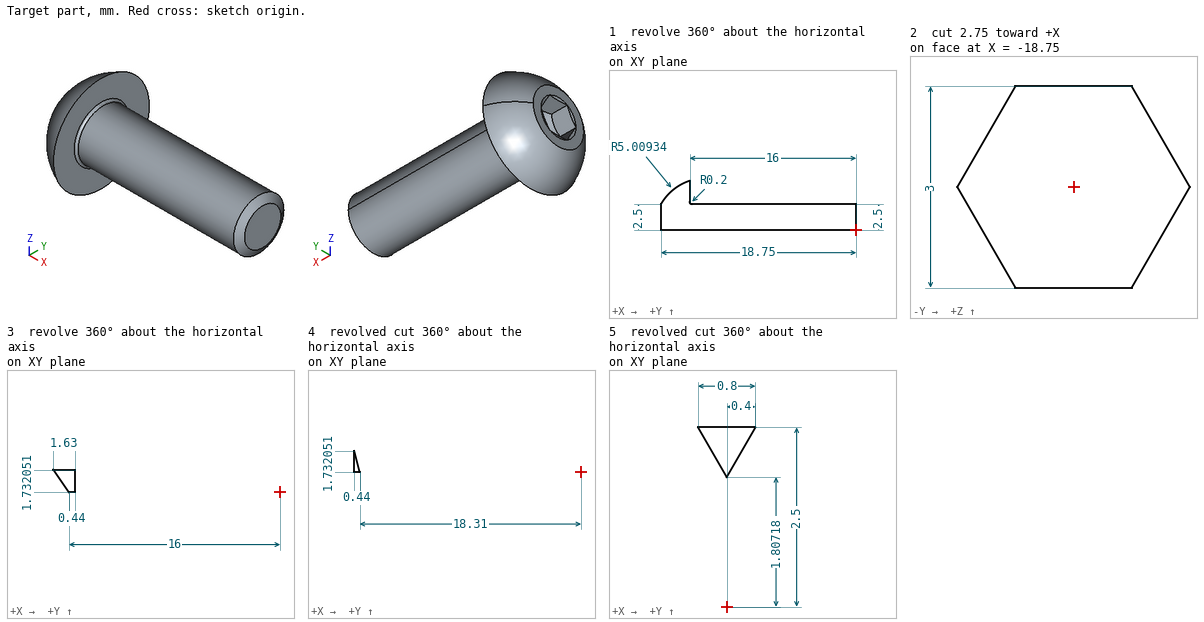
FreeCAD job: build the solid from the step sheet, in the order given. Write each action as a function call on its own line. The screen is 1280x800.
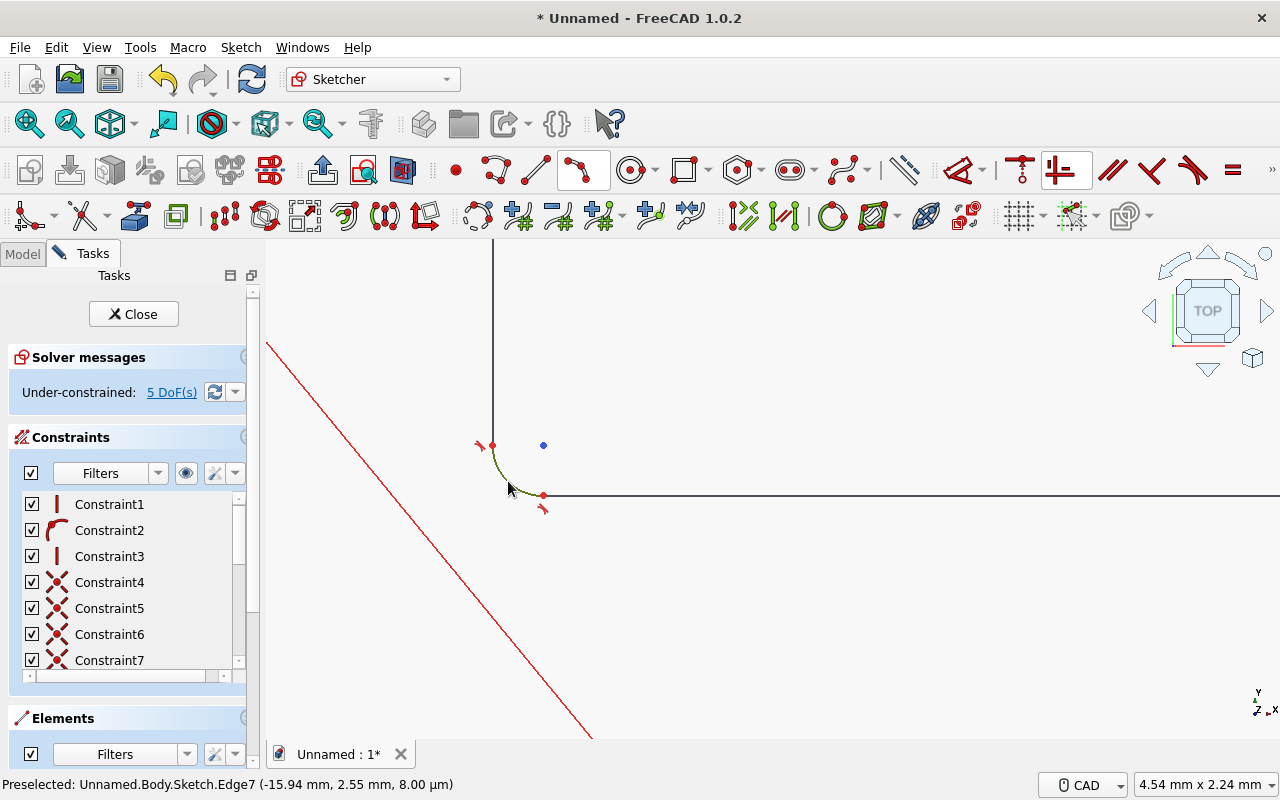
key(k)
key(r)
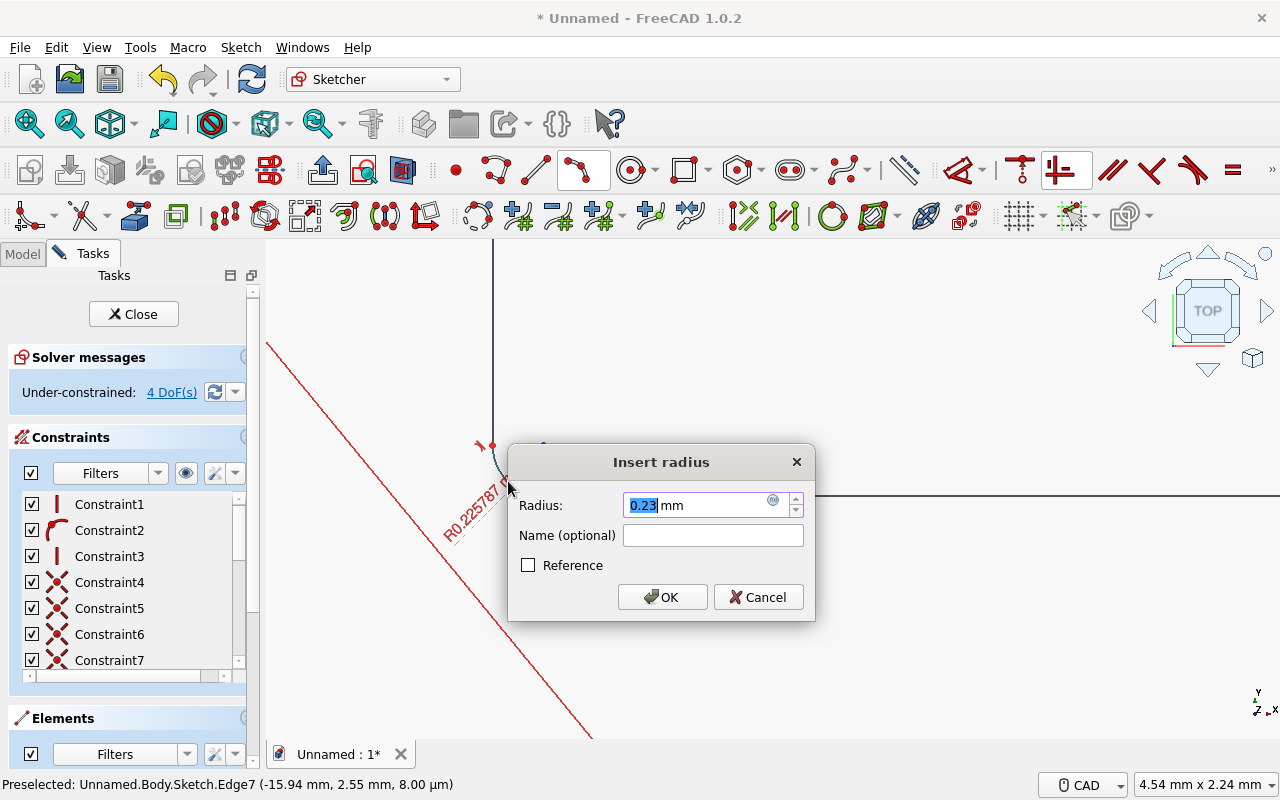
text(0.2)
key(Return)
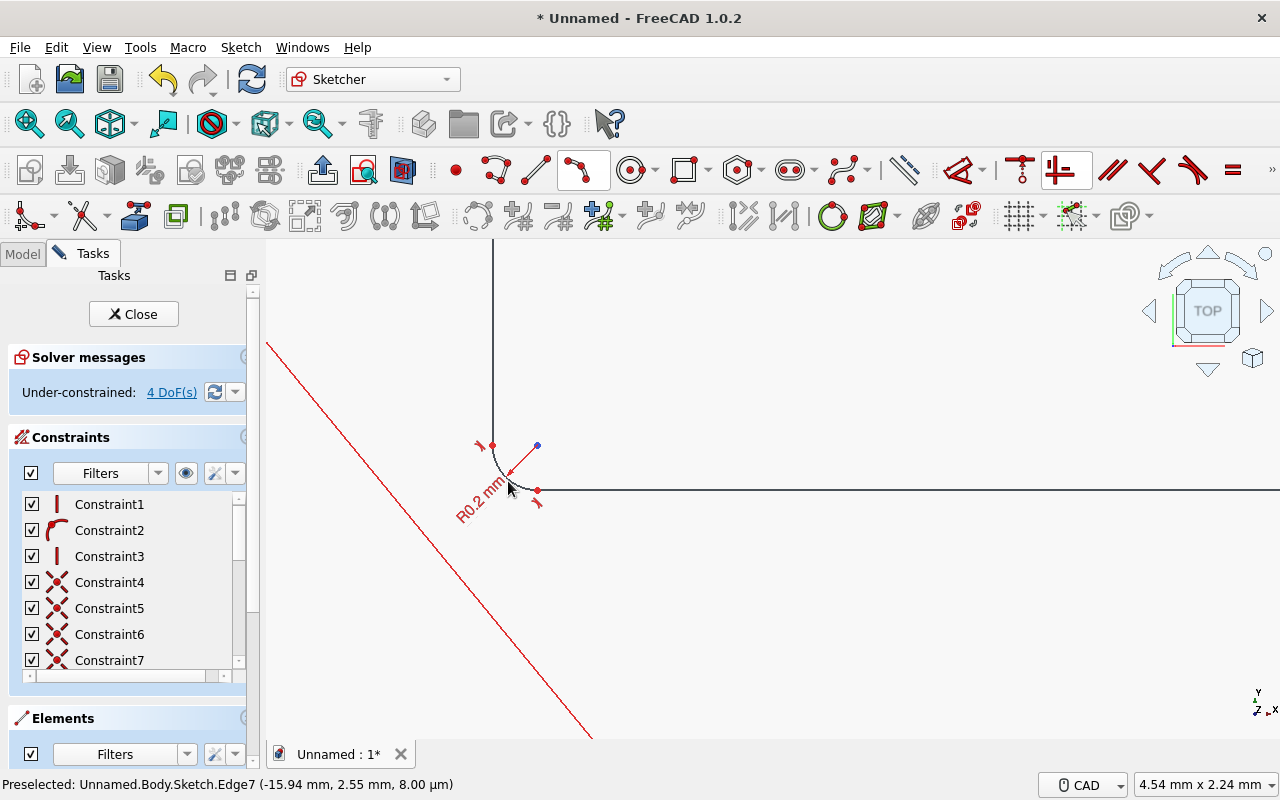
scroll(506, 484, down, 10)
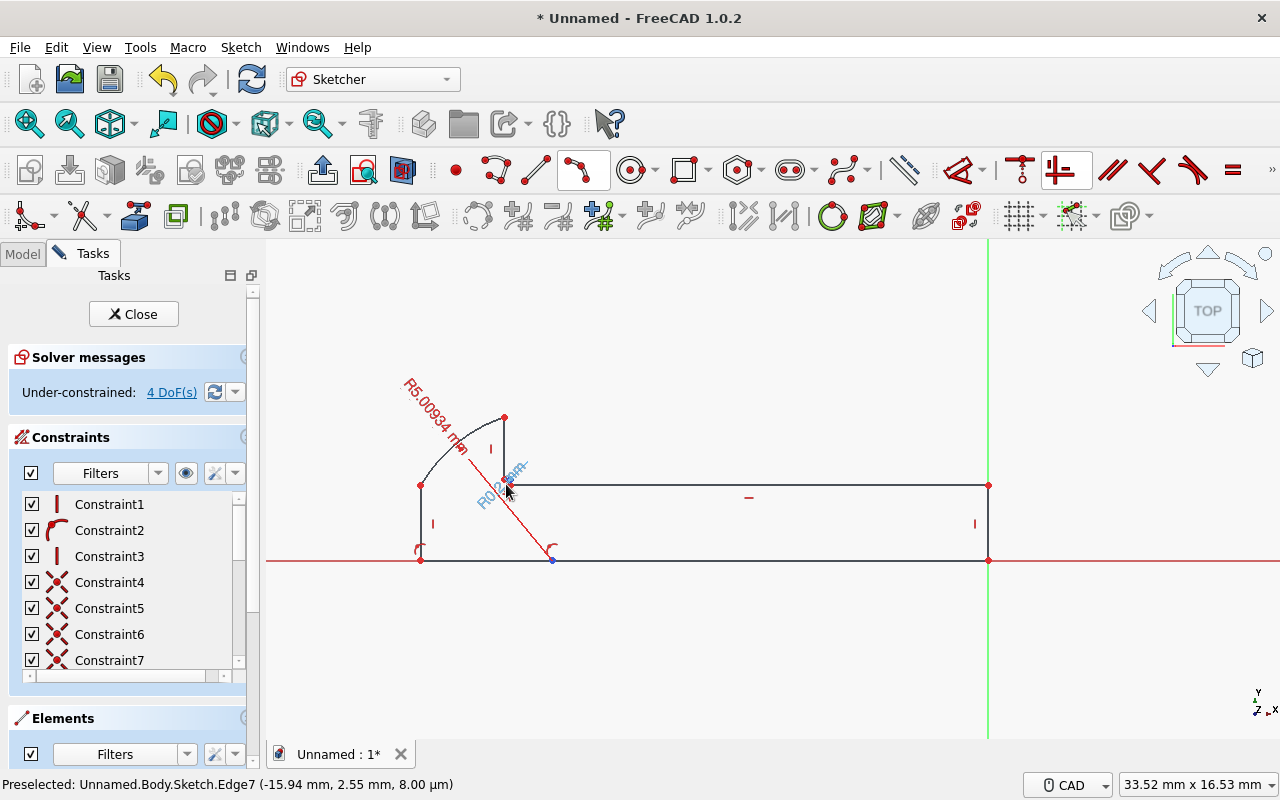
click(421, 508)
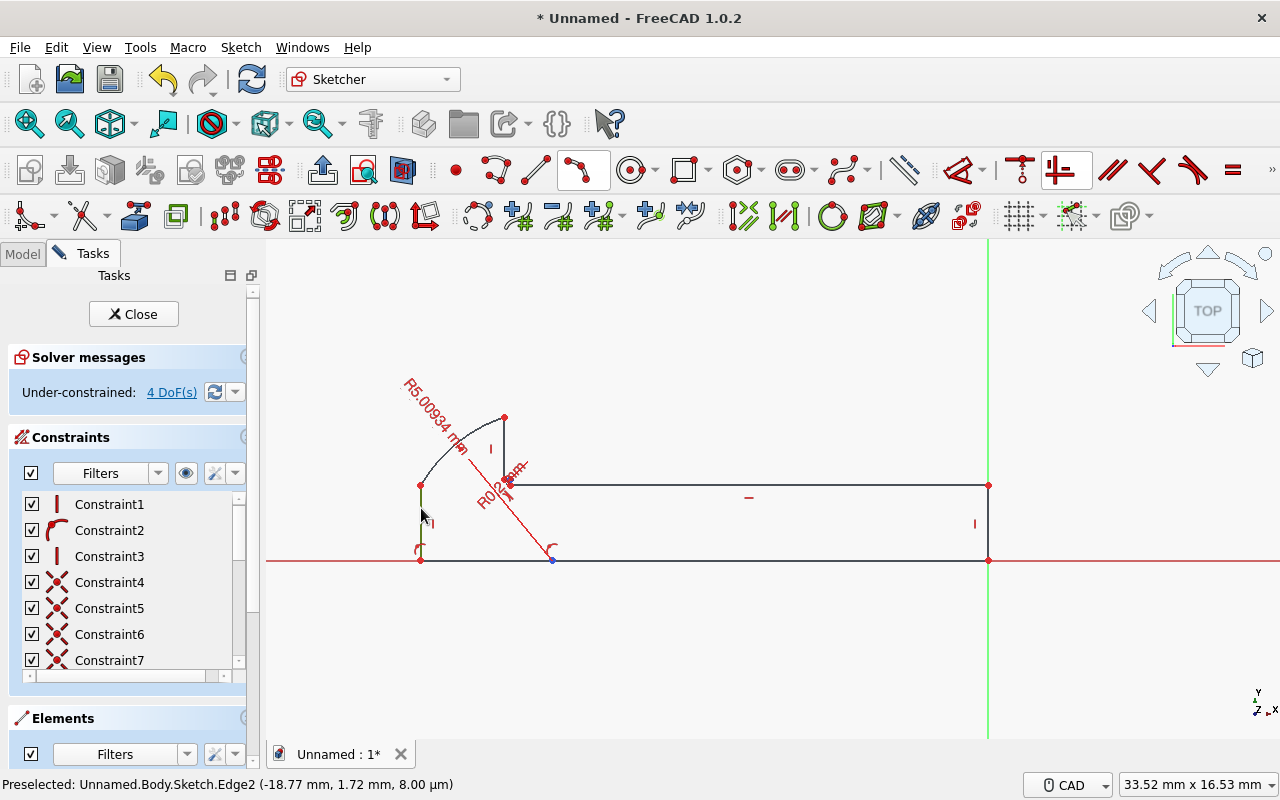
key(i)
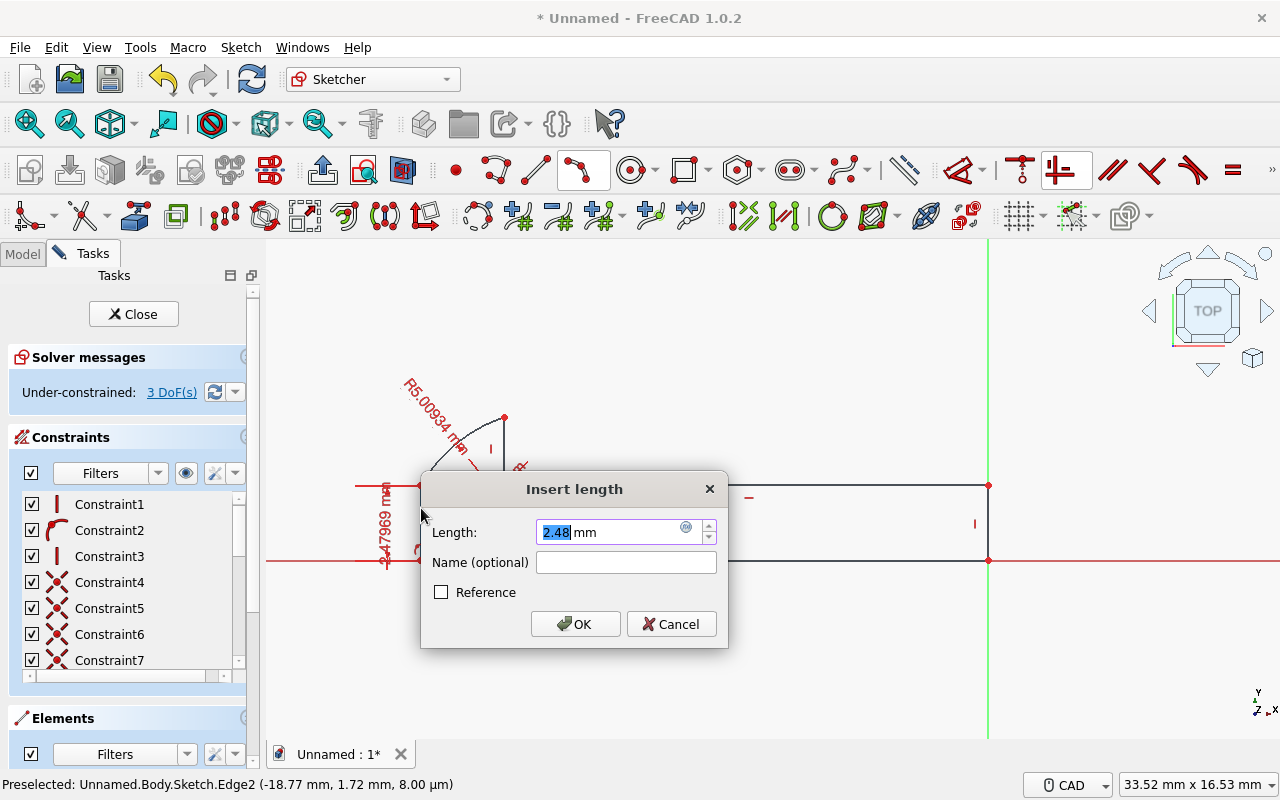
text(2.5)
key(Return)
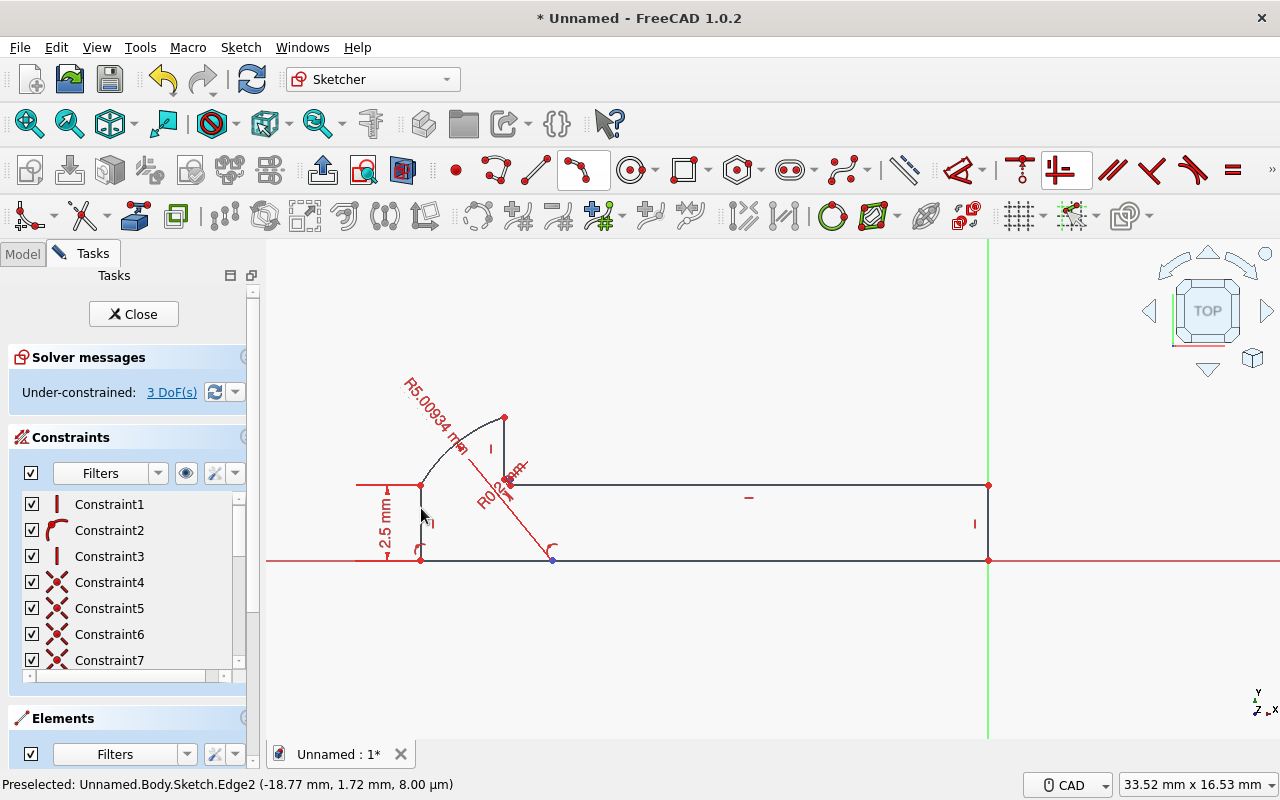
click(988, 538)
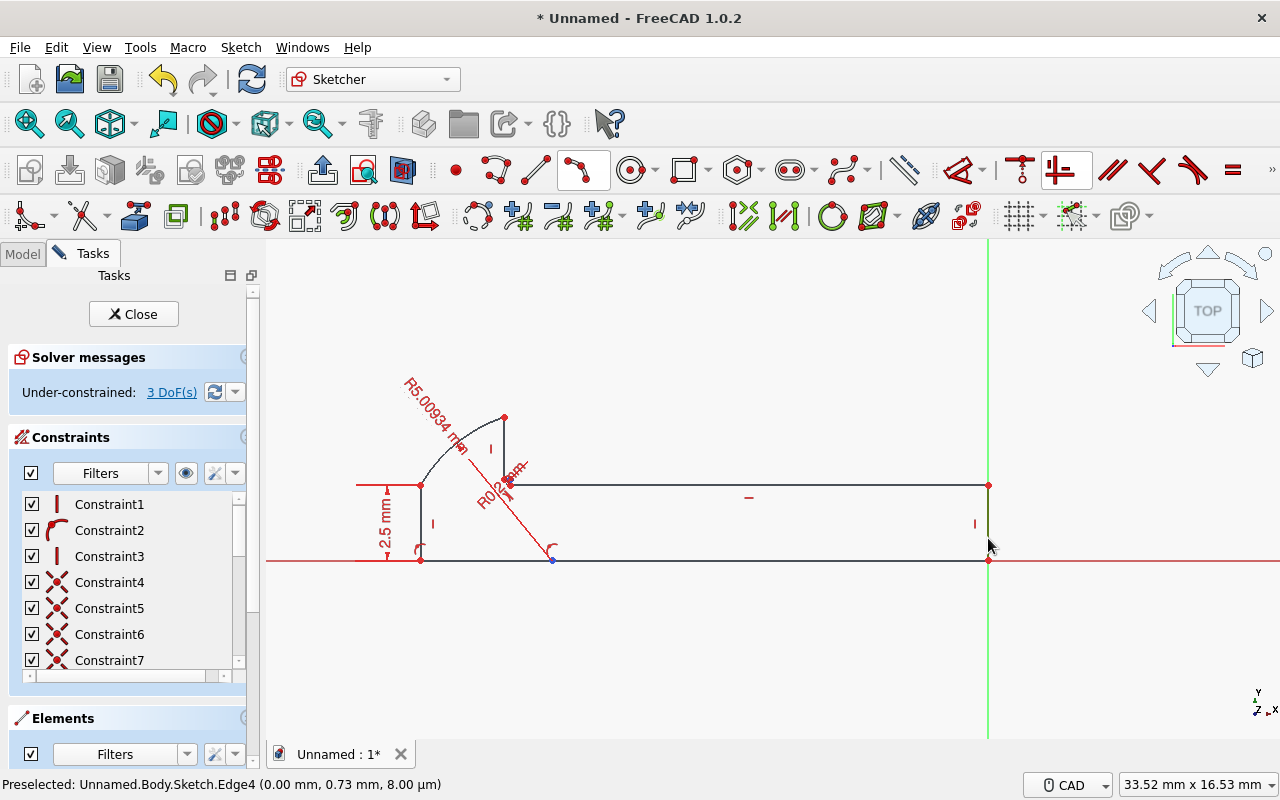
click(984, 170)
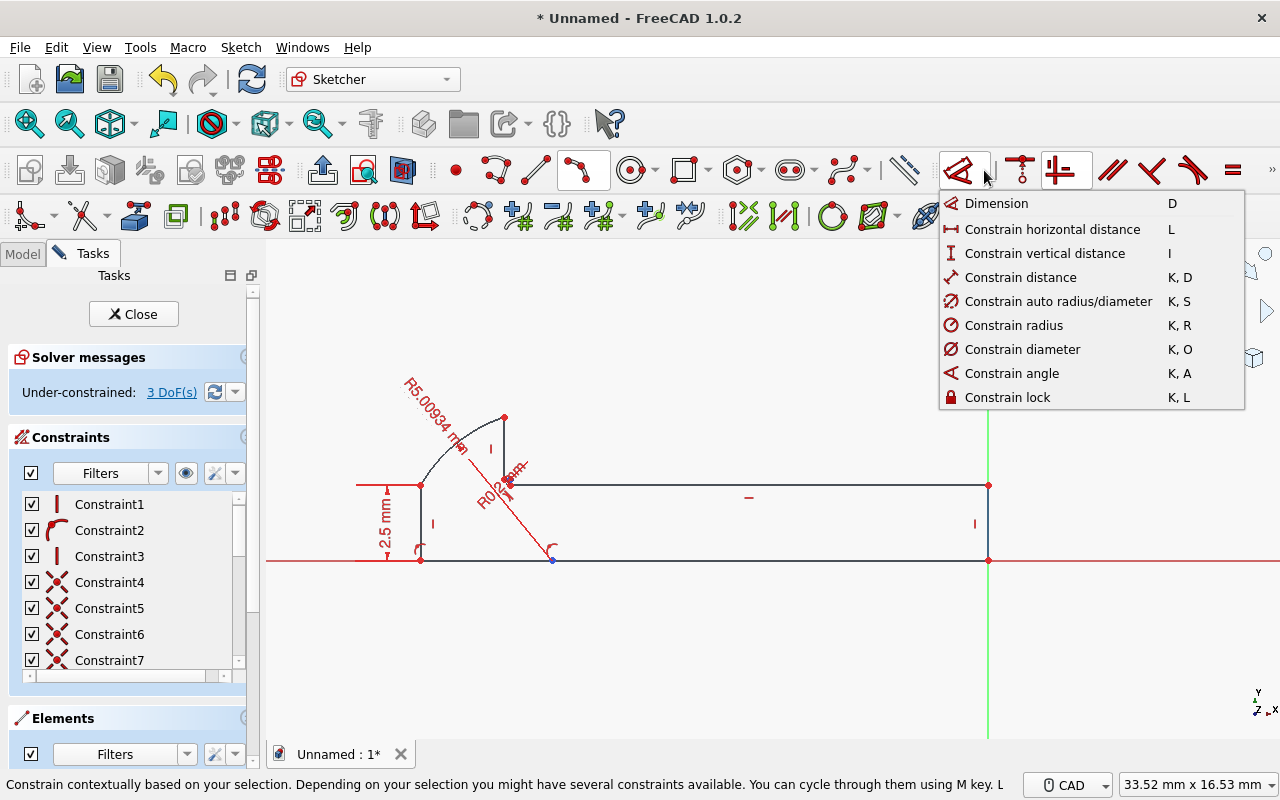
click(1092, 253)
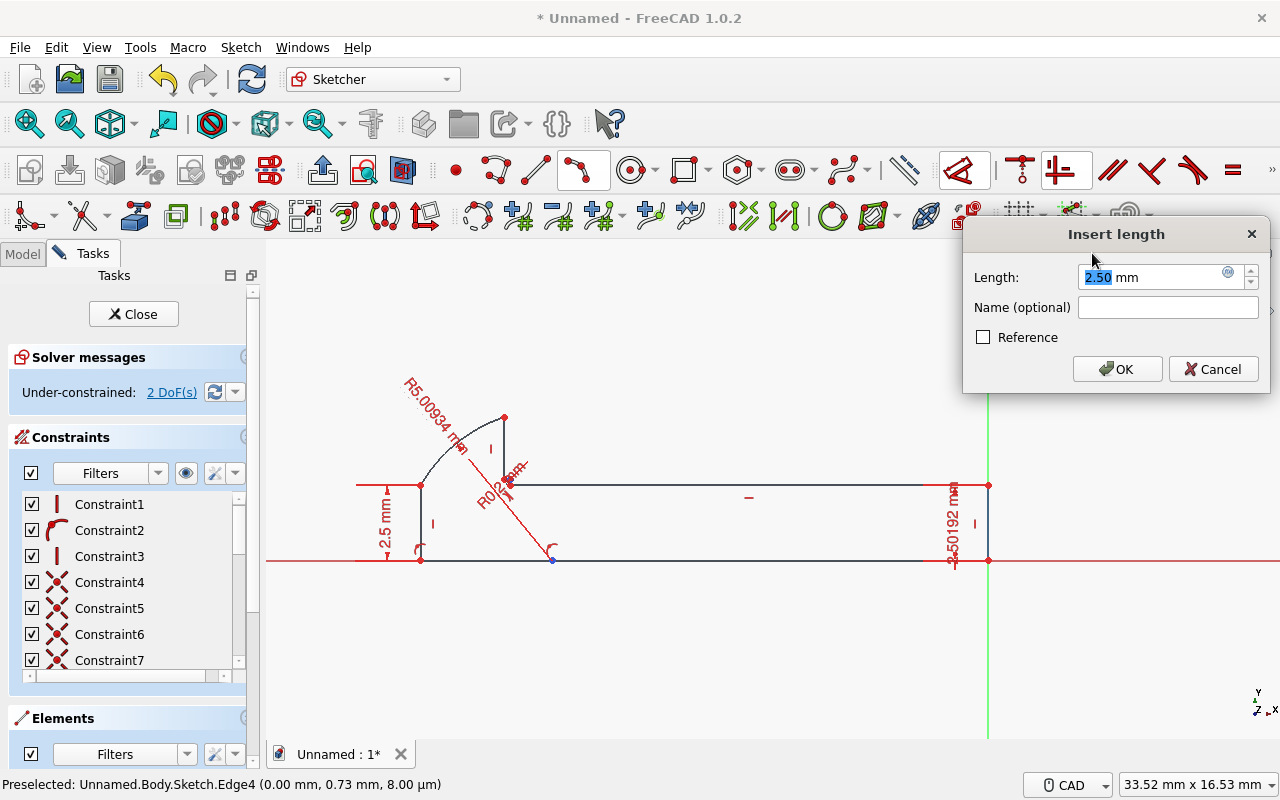
text(2.5)
key(Return)